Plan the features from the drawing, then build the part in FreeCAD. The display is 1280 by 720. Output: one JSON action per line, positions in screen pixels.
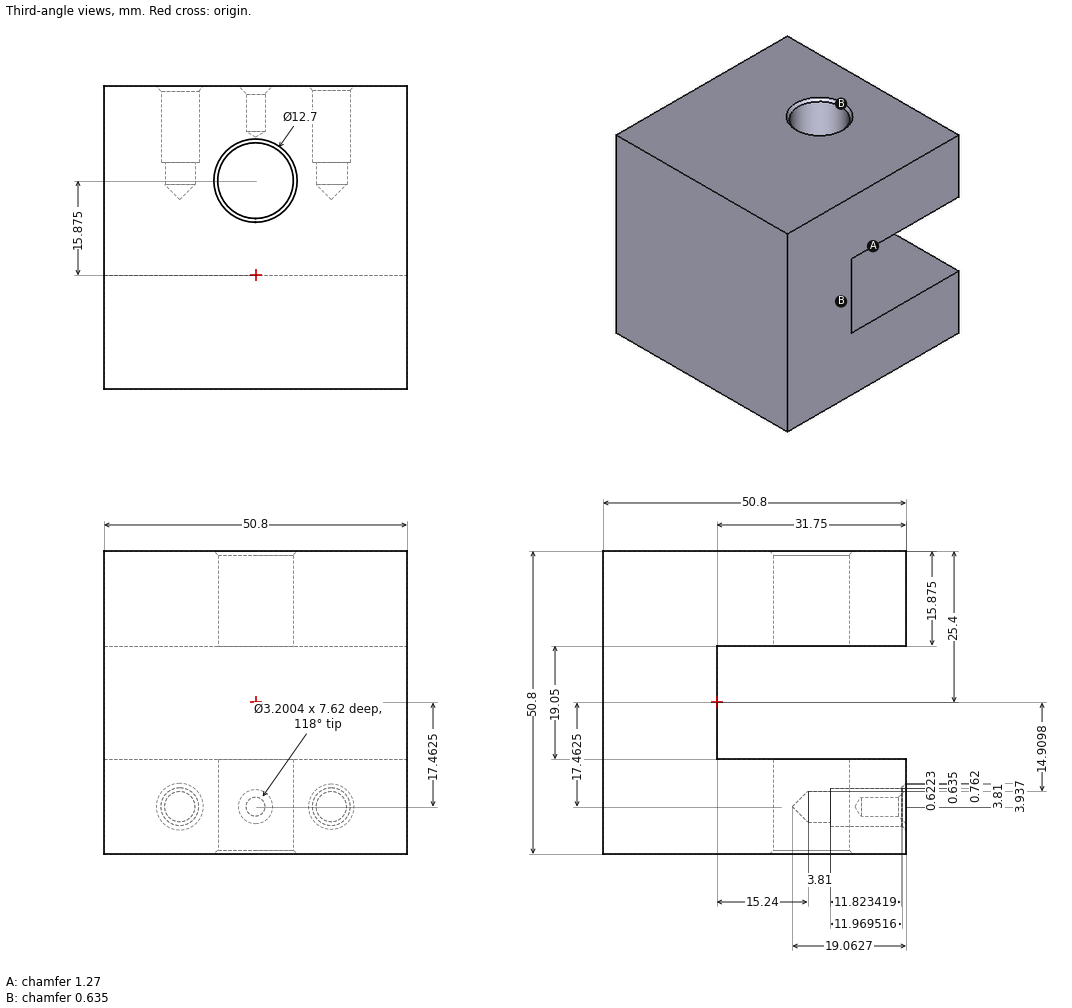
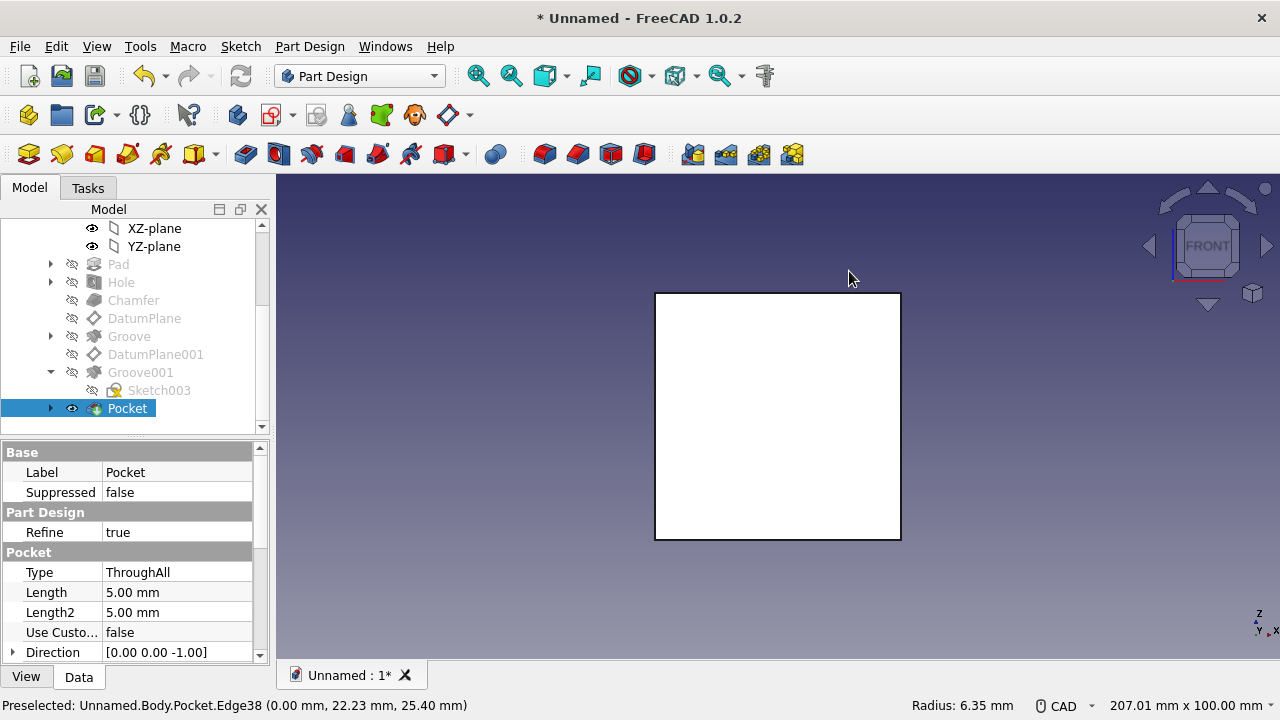
{"action": "key", "text": "3"}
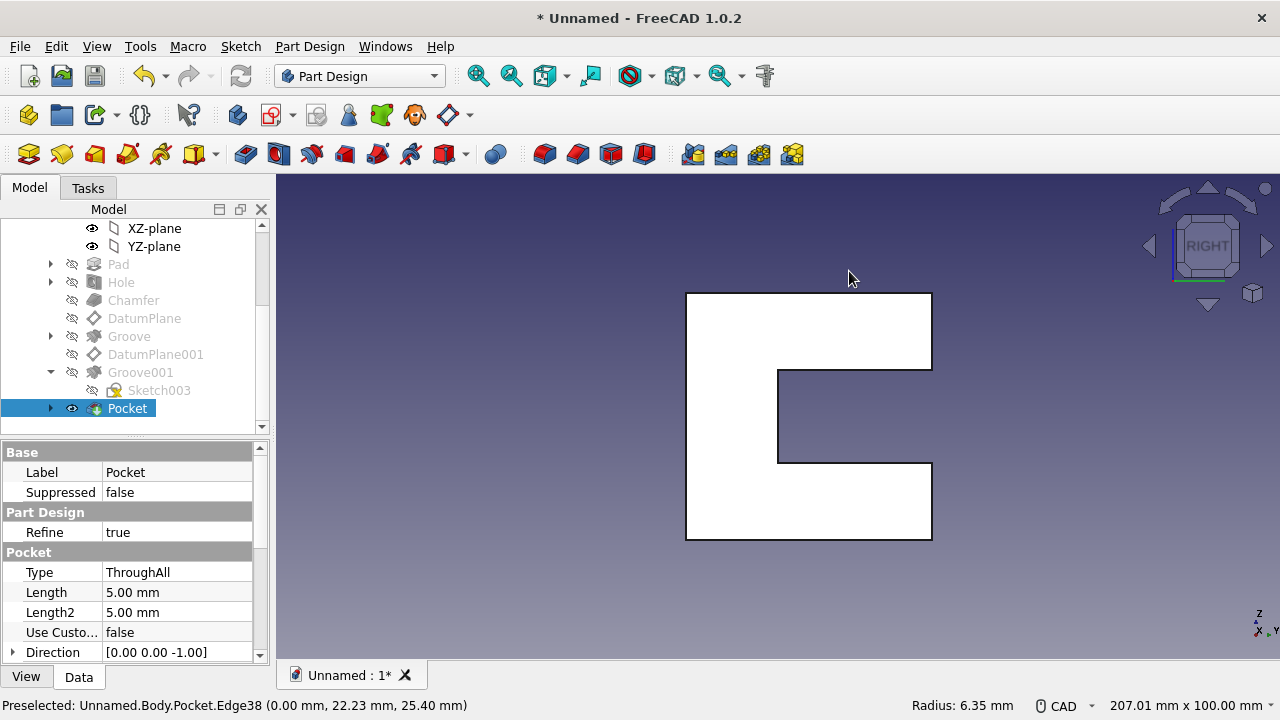
{"action": "key", "text": "5"}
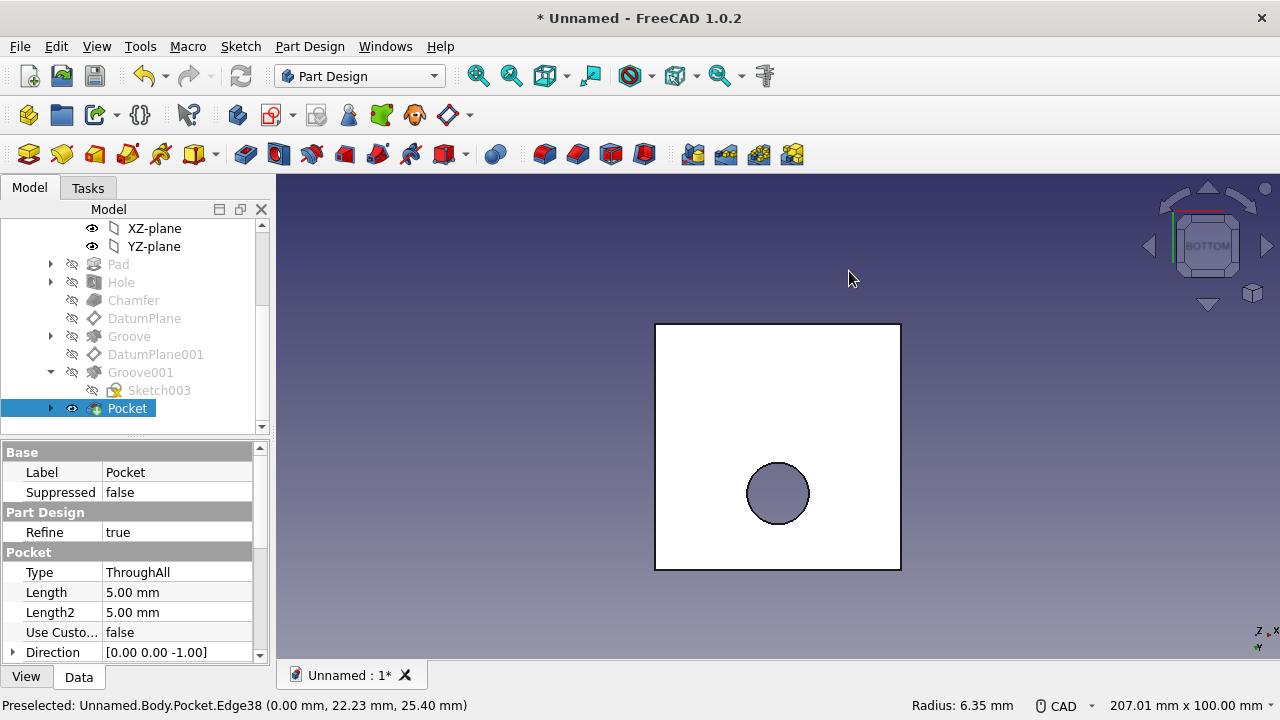
{"action": "left_click", "coordinate": [778, 523], "text": "ctrl"}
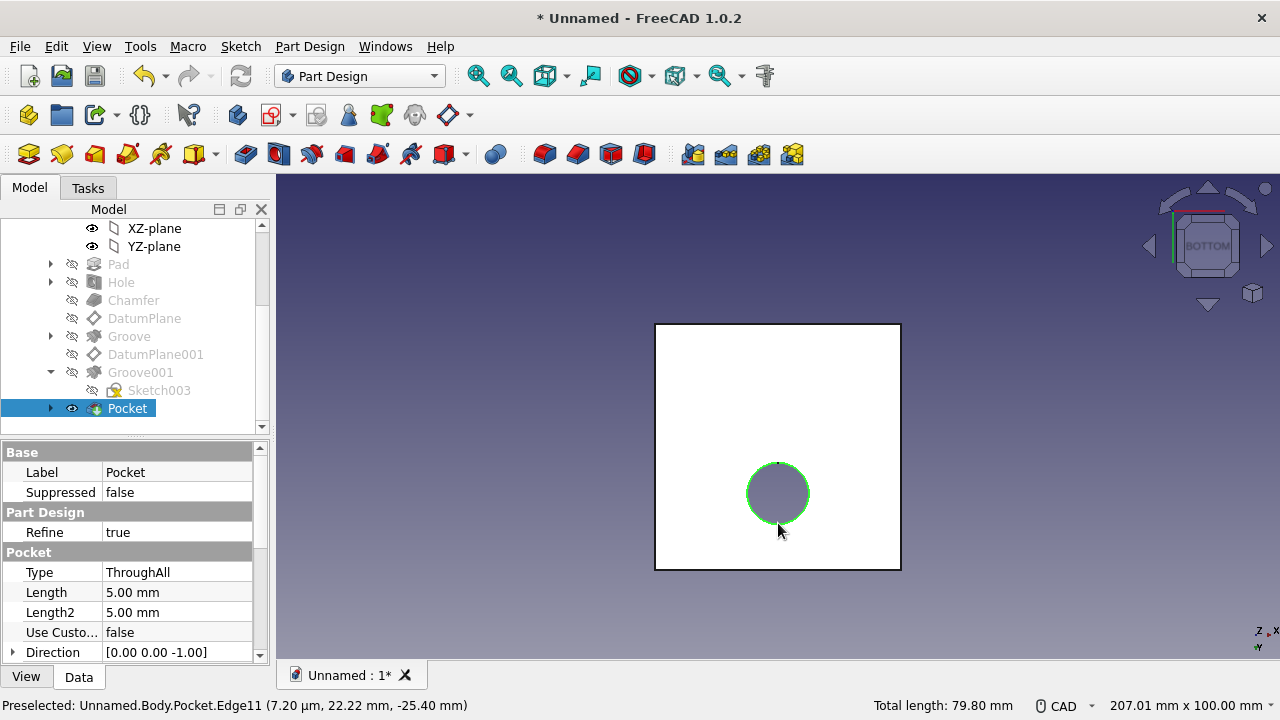
{"action": "left_click", "coordinate": [578, 154]}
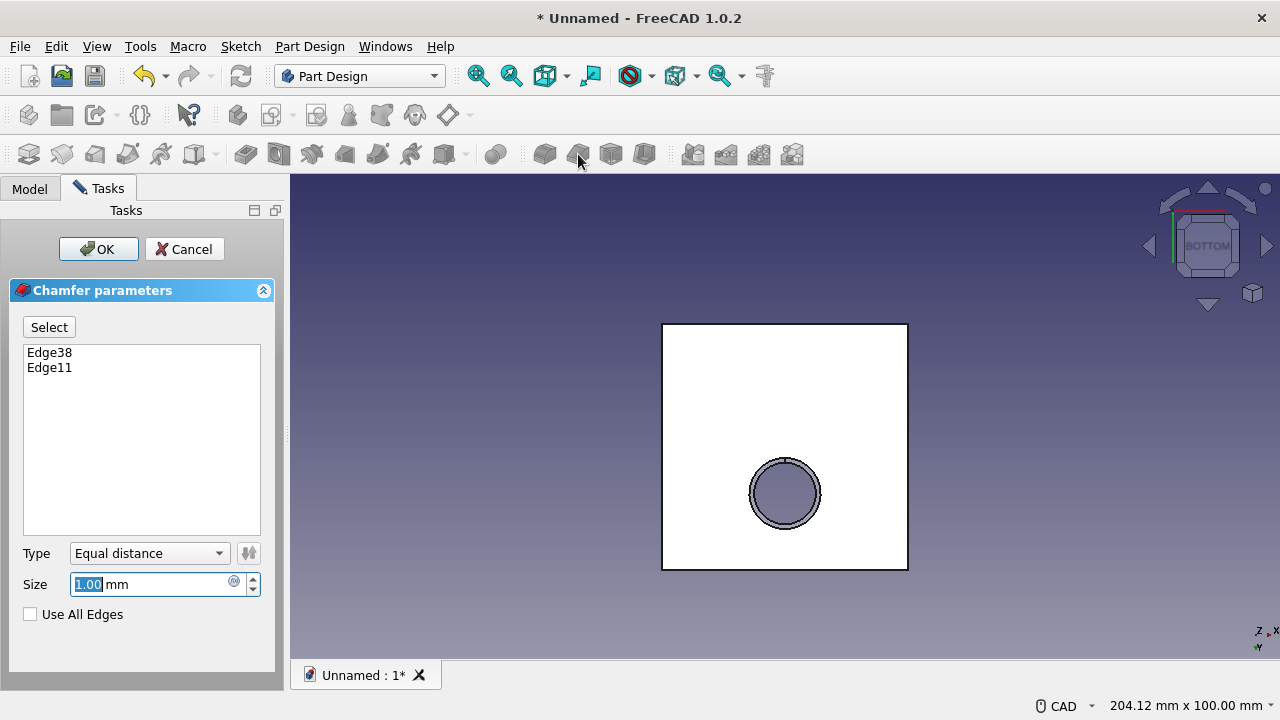
{"action": "type", "text": "0.635"}
{"action": "key", "text": "Tab"}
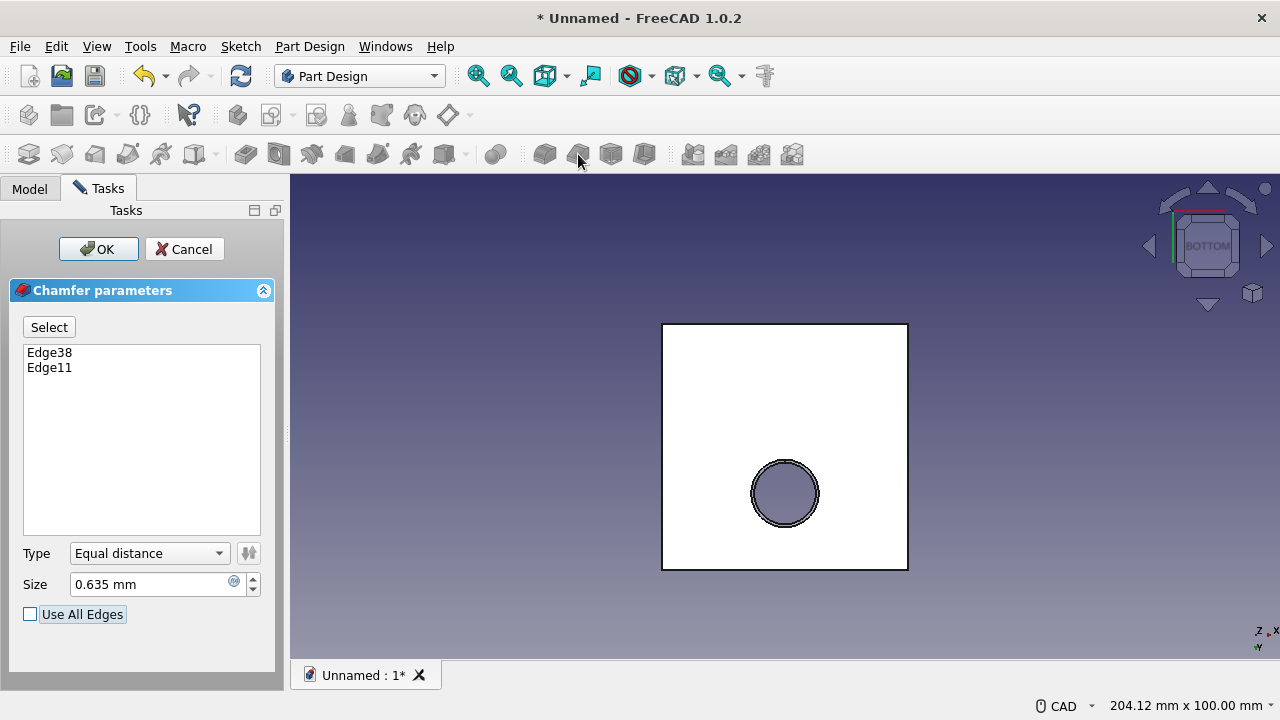
{"action": "left_click", "coordinate": [99, 249]}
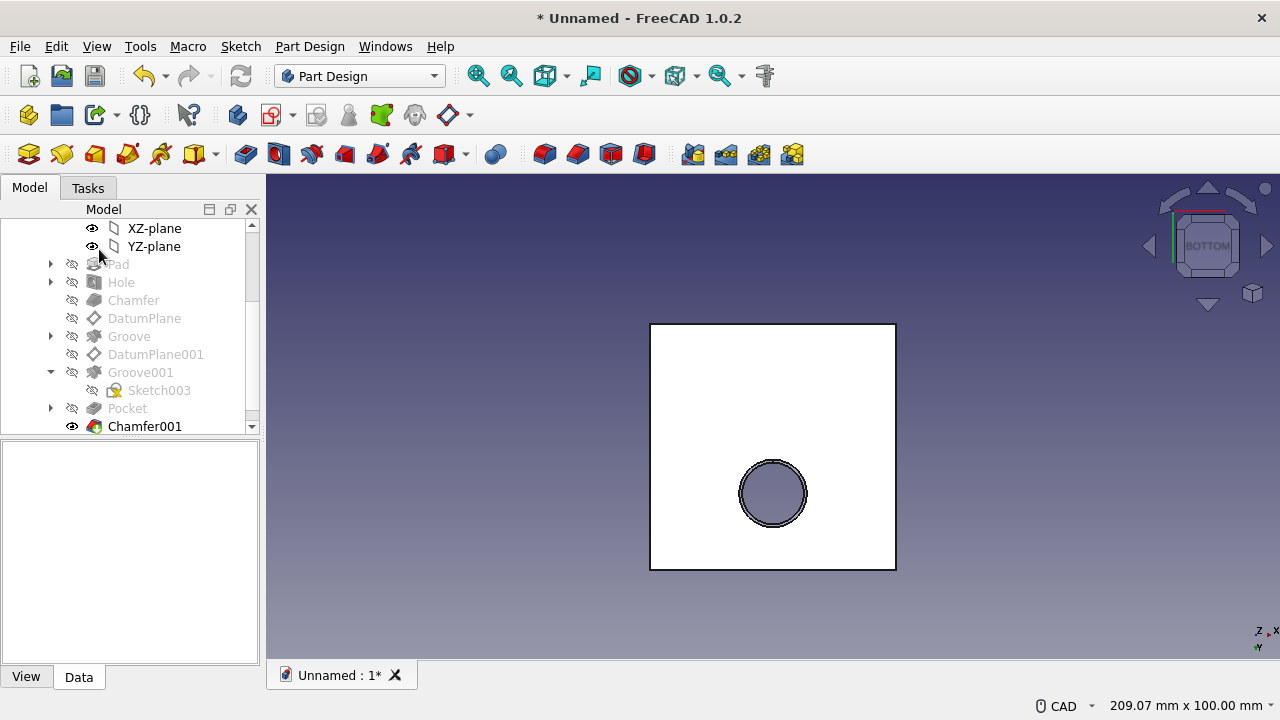
{"action": "key", "text": "0"}